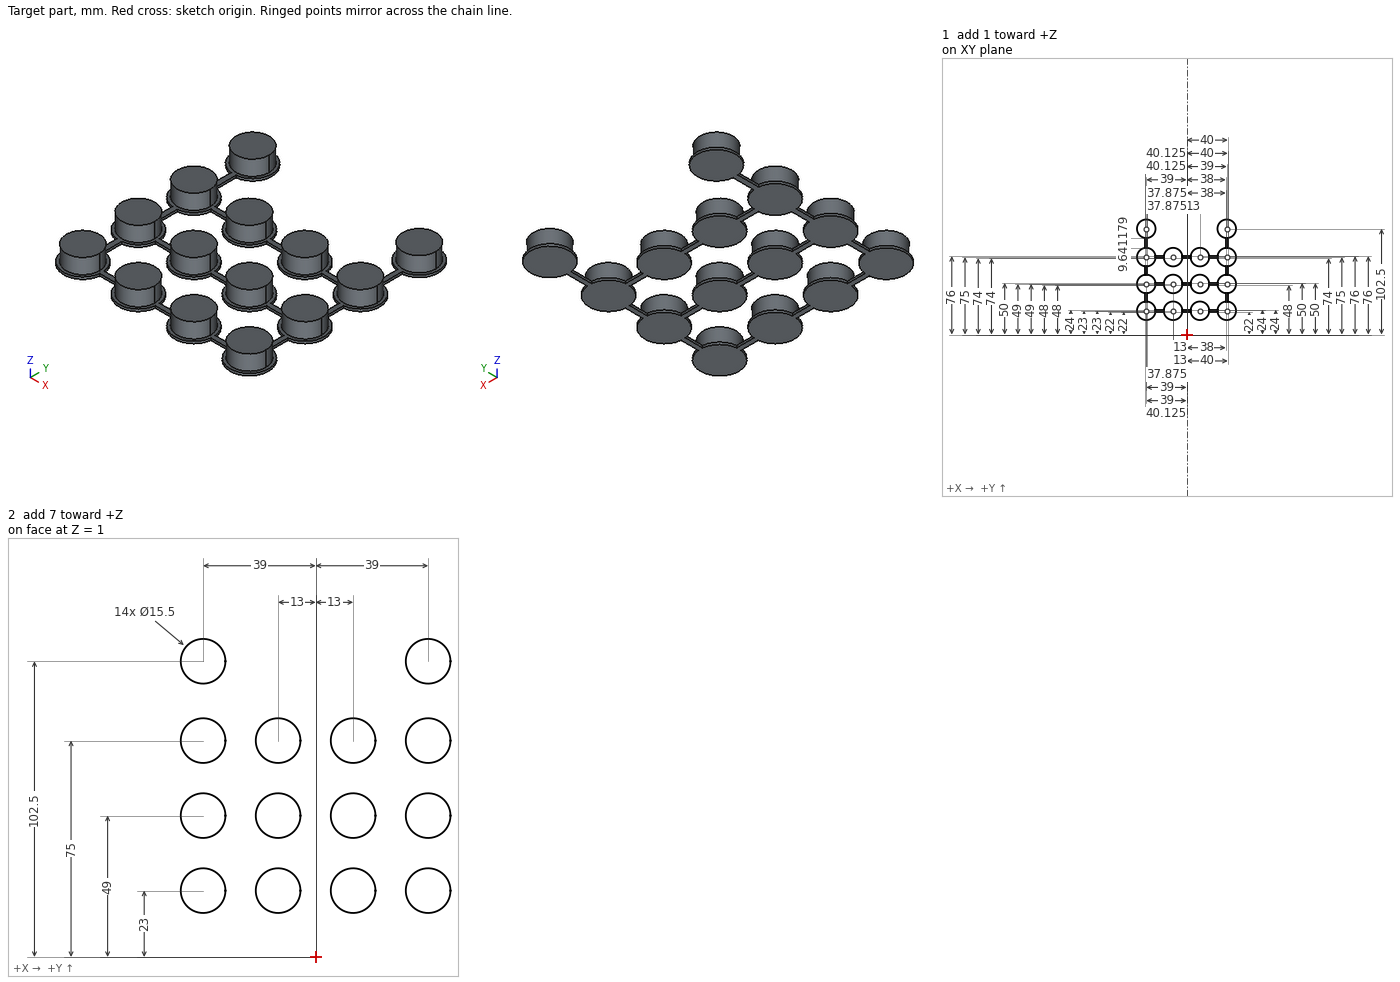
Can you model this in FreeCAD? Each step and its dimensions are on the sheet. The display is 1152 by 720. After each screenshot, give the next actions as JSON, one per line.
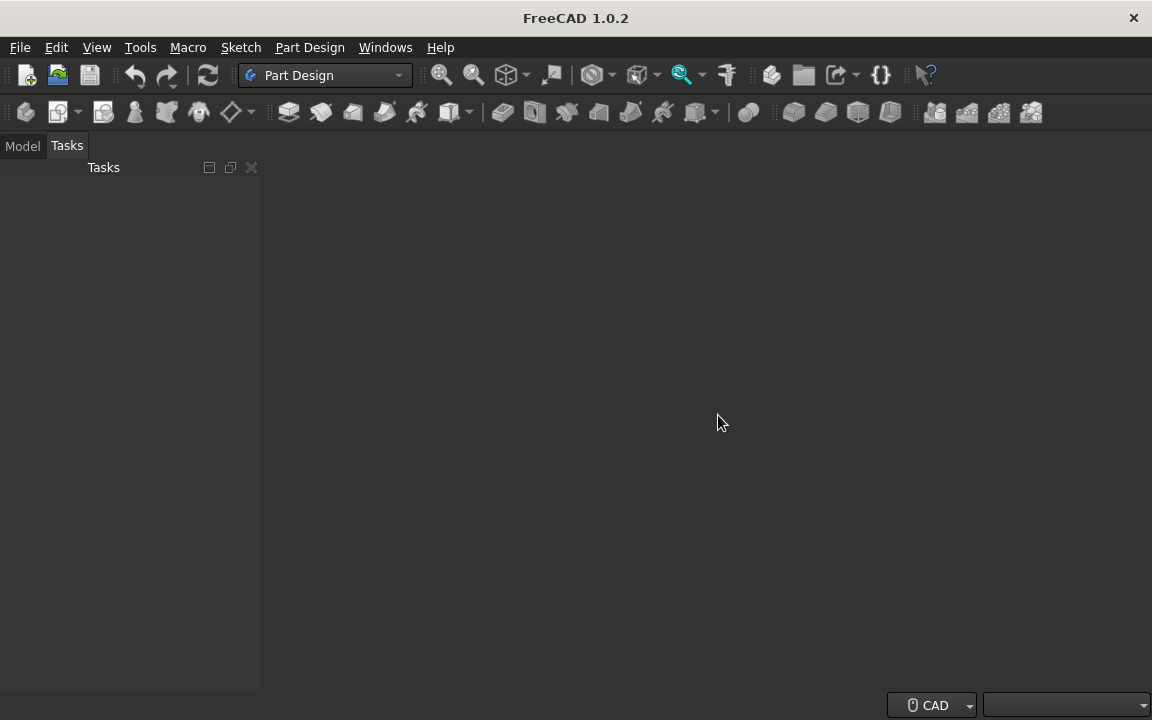
{"action": "left_click", "coordinate": [26, 76]}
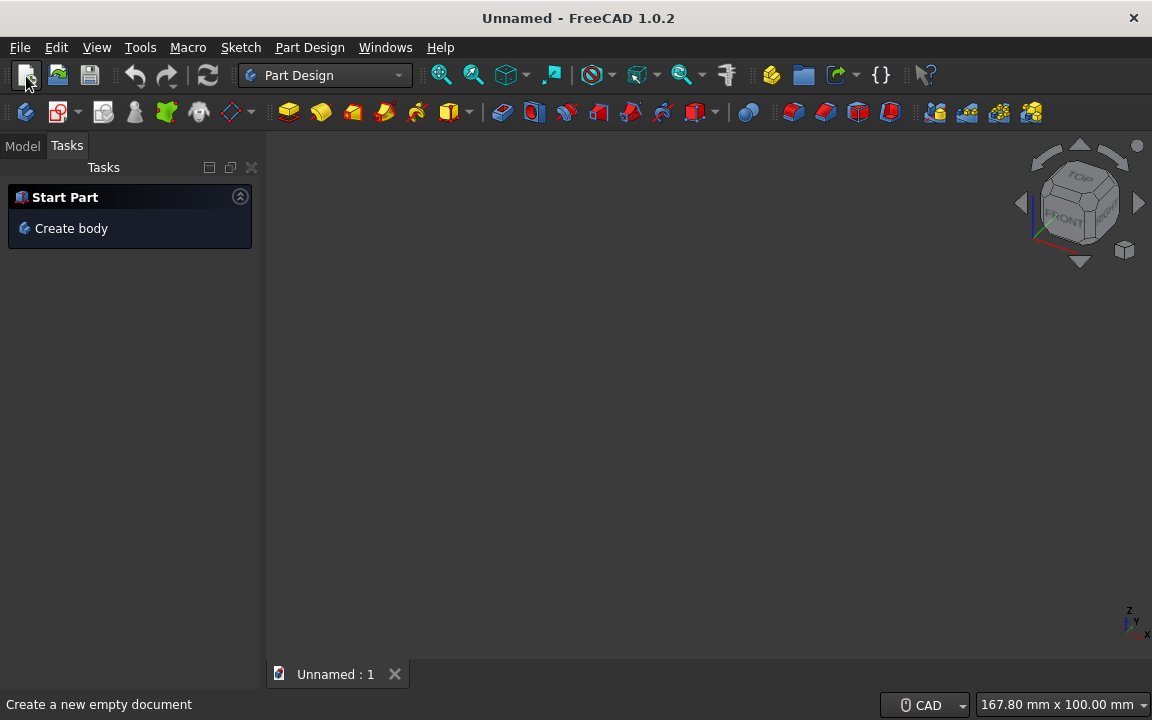
{"action": "left_click", "coordinate": [58, 112]}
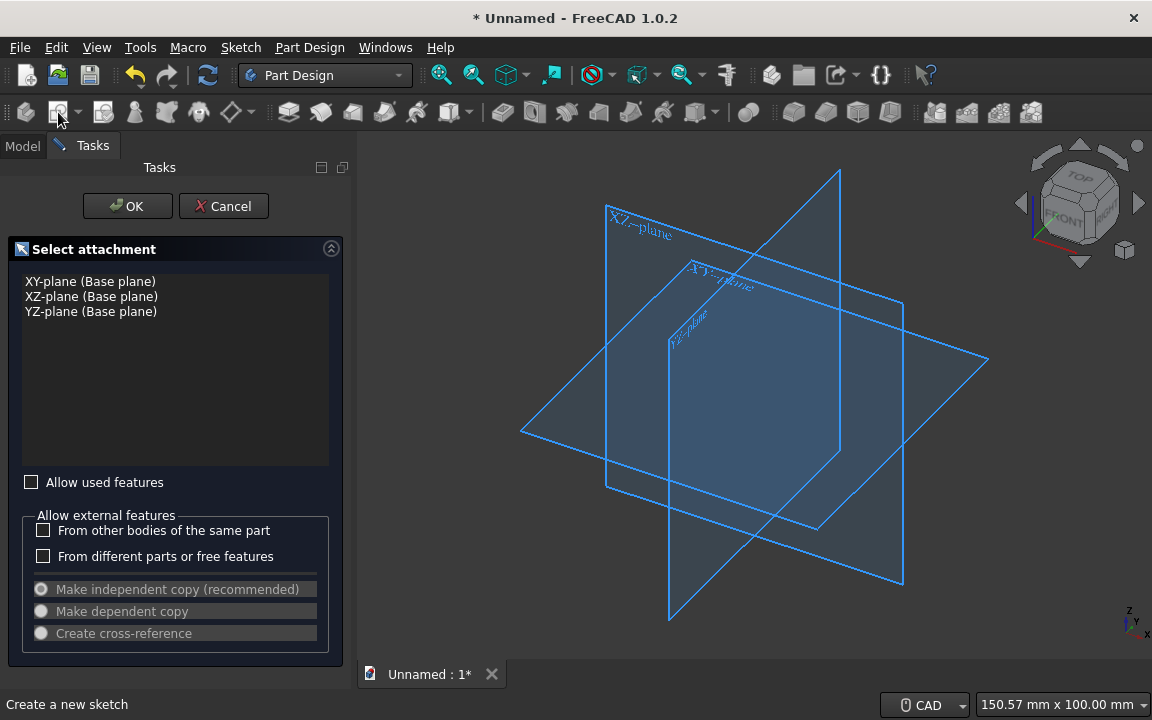
{"action": "left_click", "coordinate": [82, 282]}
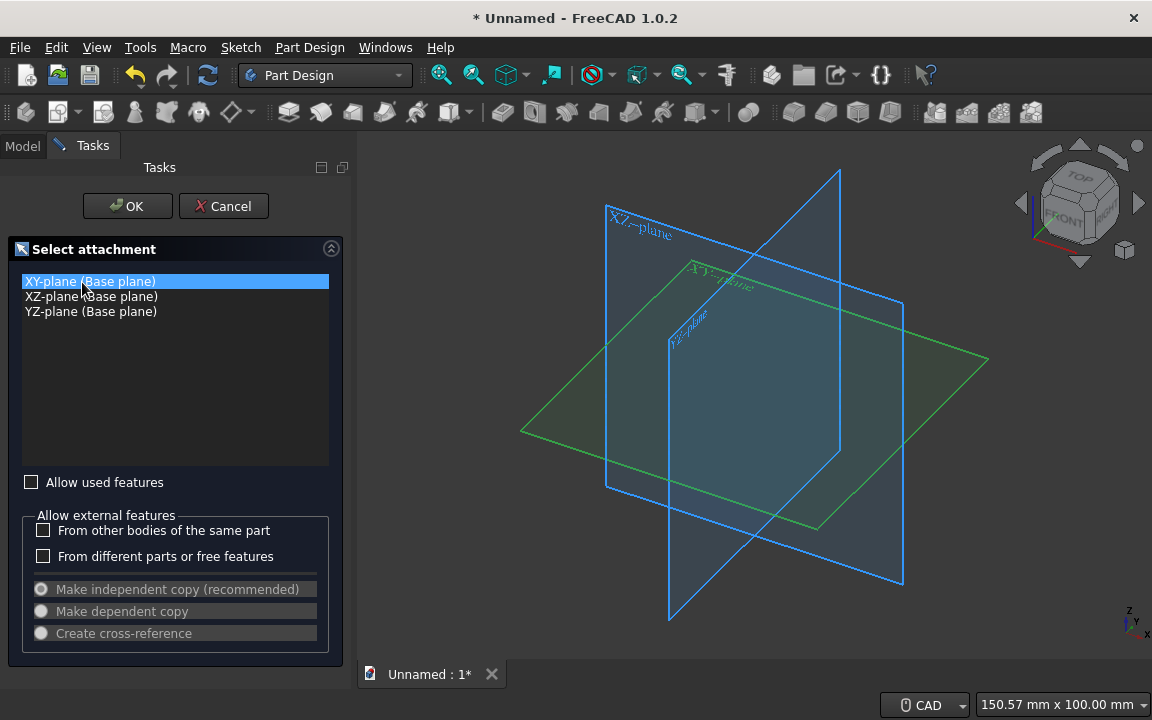
{"action": "left_click", "coordinate": [128, 206]}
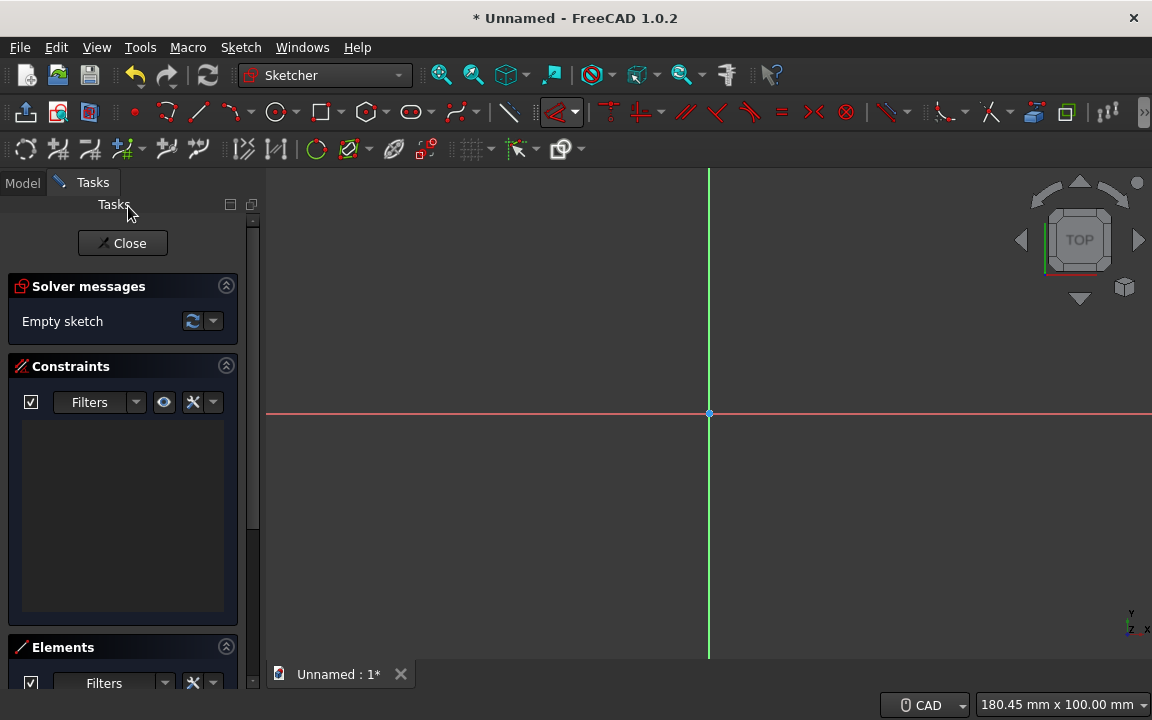
{"action": "scroll", "coordinate": [585, 631], "scroll_direction": "down", "scroll_amount": 4}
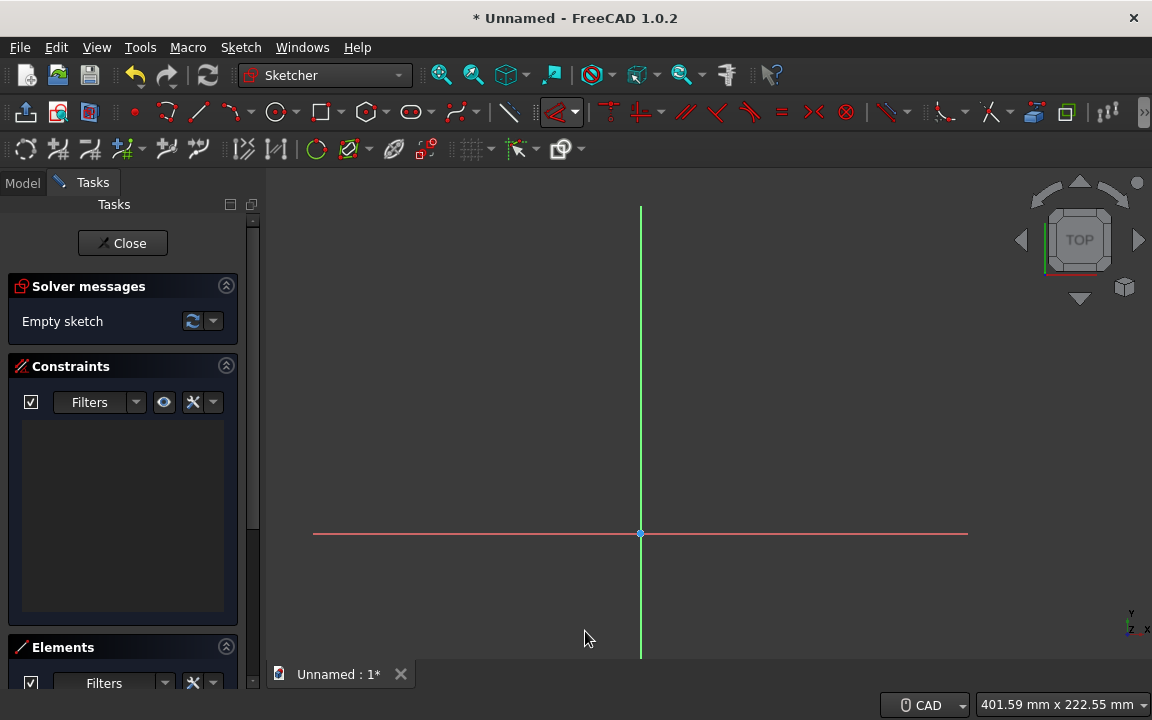
{"action": "left_click", "coordinate": [200, 112]}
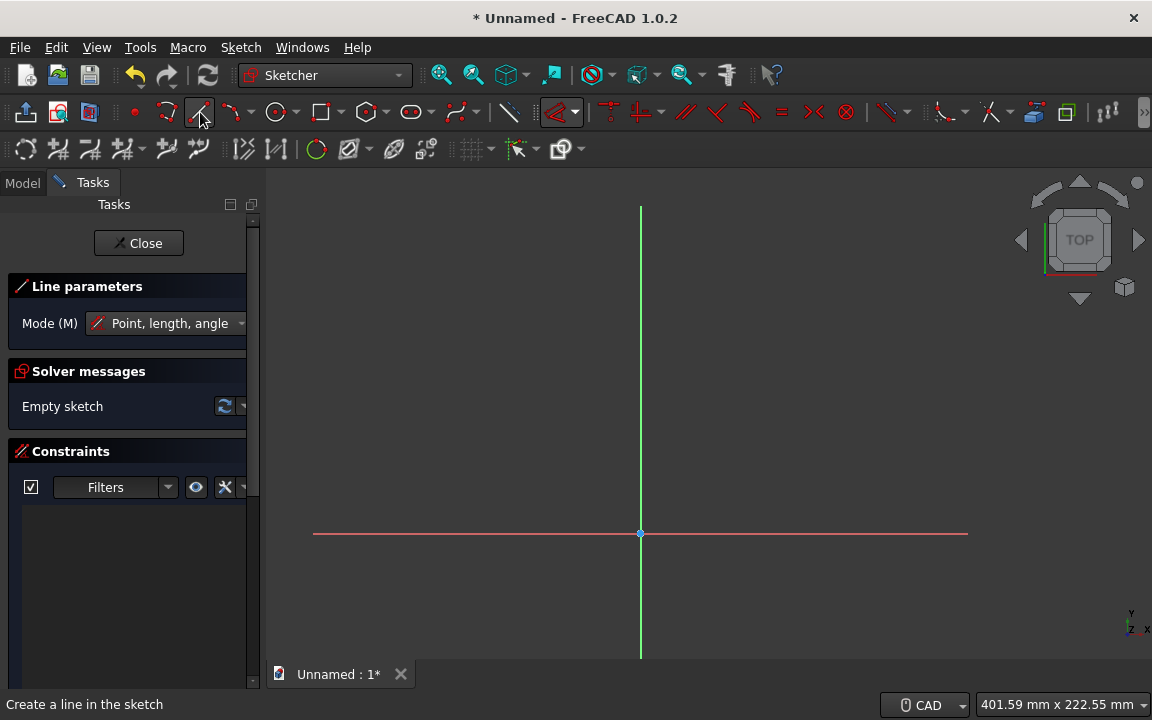
{"action": "left_click", "coordinate": [552, 327]}
{"action": "left_click", "coordinate": [552, 349]}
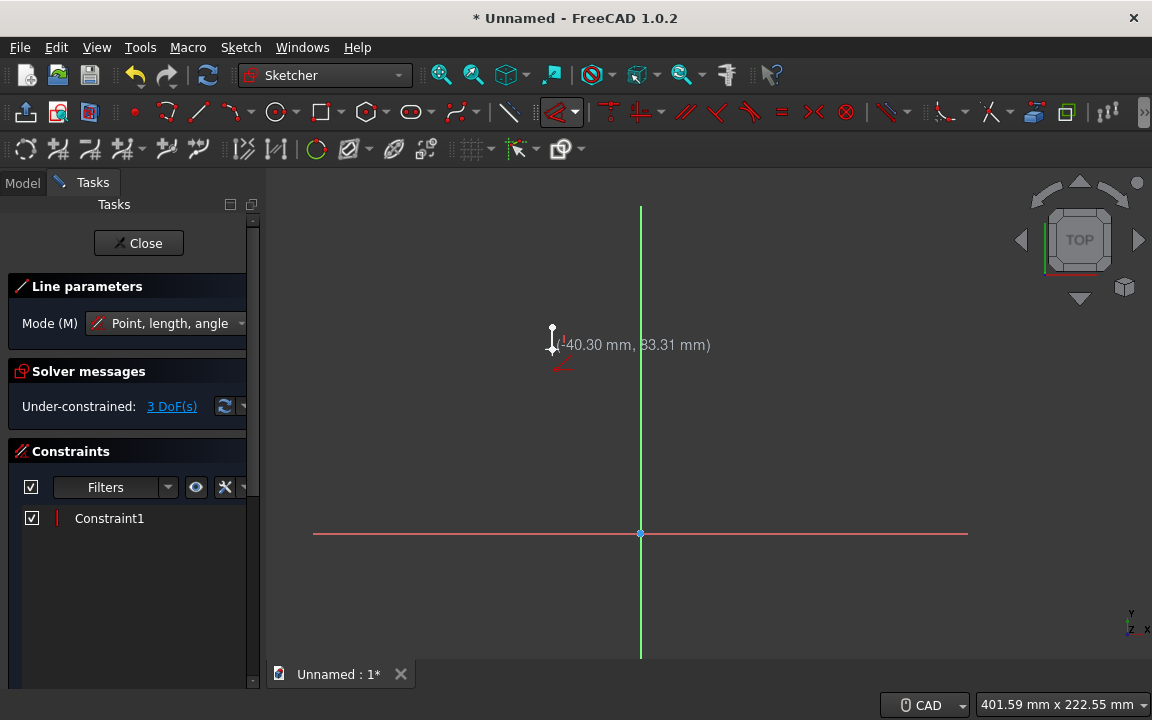
{"action": "left_click", "coordinate": [552, 388]}
{"action": "left_click", "coordinate": [552, 406]}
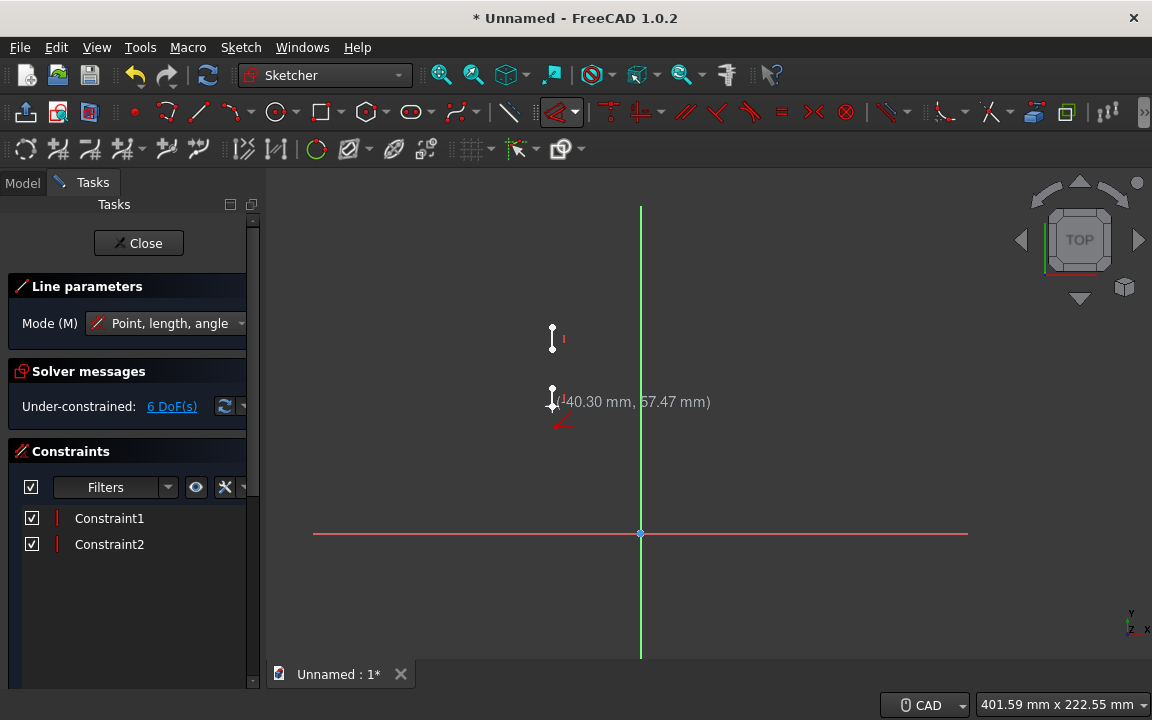
{"action": "left_click", "coordinate": [552, 445]}
{"action": "left_click", "coordinate": [552, 463]}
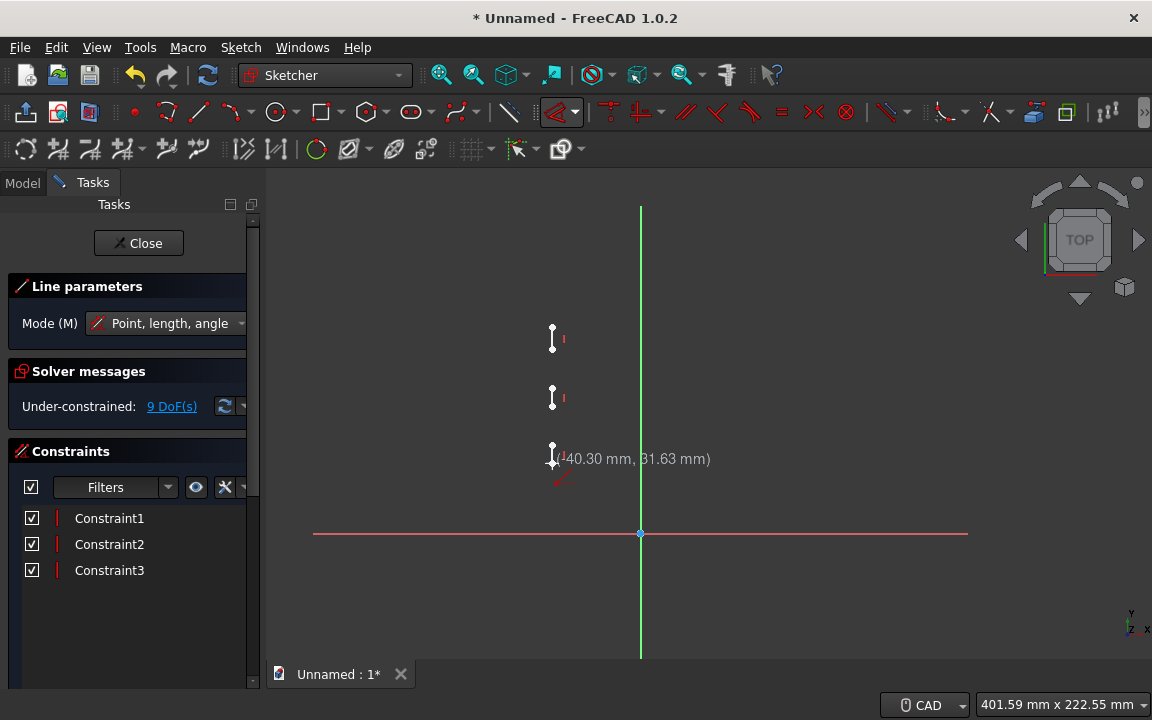
{"action": "left_click", "coordinate": [575, 485]}
{"action": "left_click", "coordinate": [593, 485]}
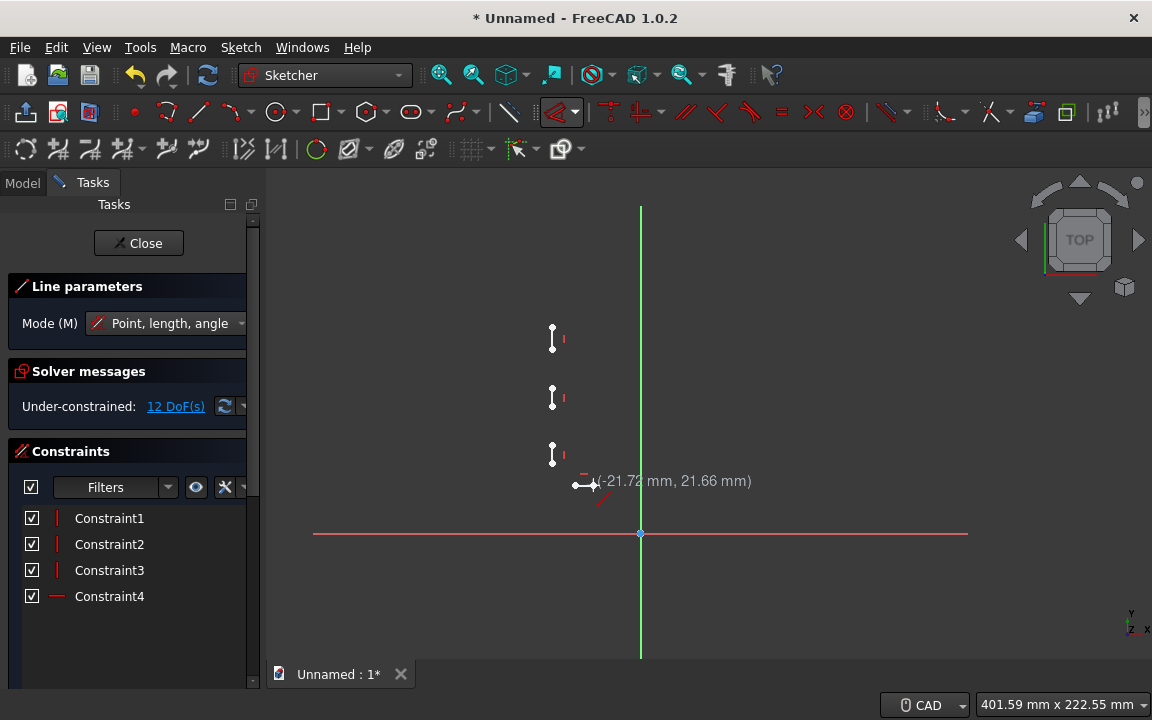
{"action": "scroll", "coordinate": [632, 485], "scroll_direction": "up", "scroll_amount": 3}